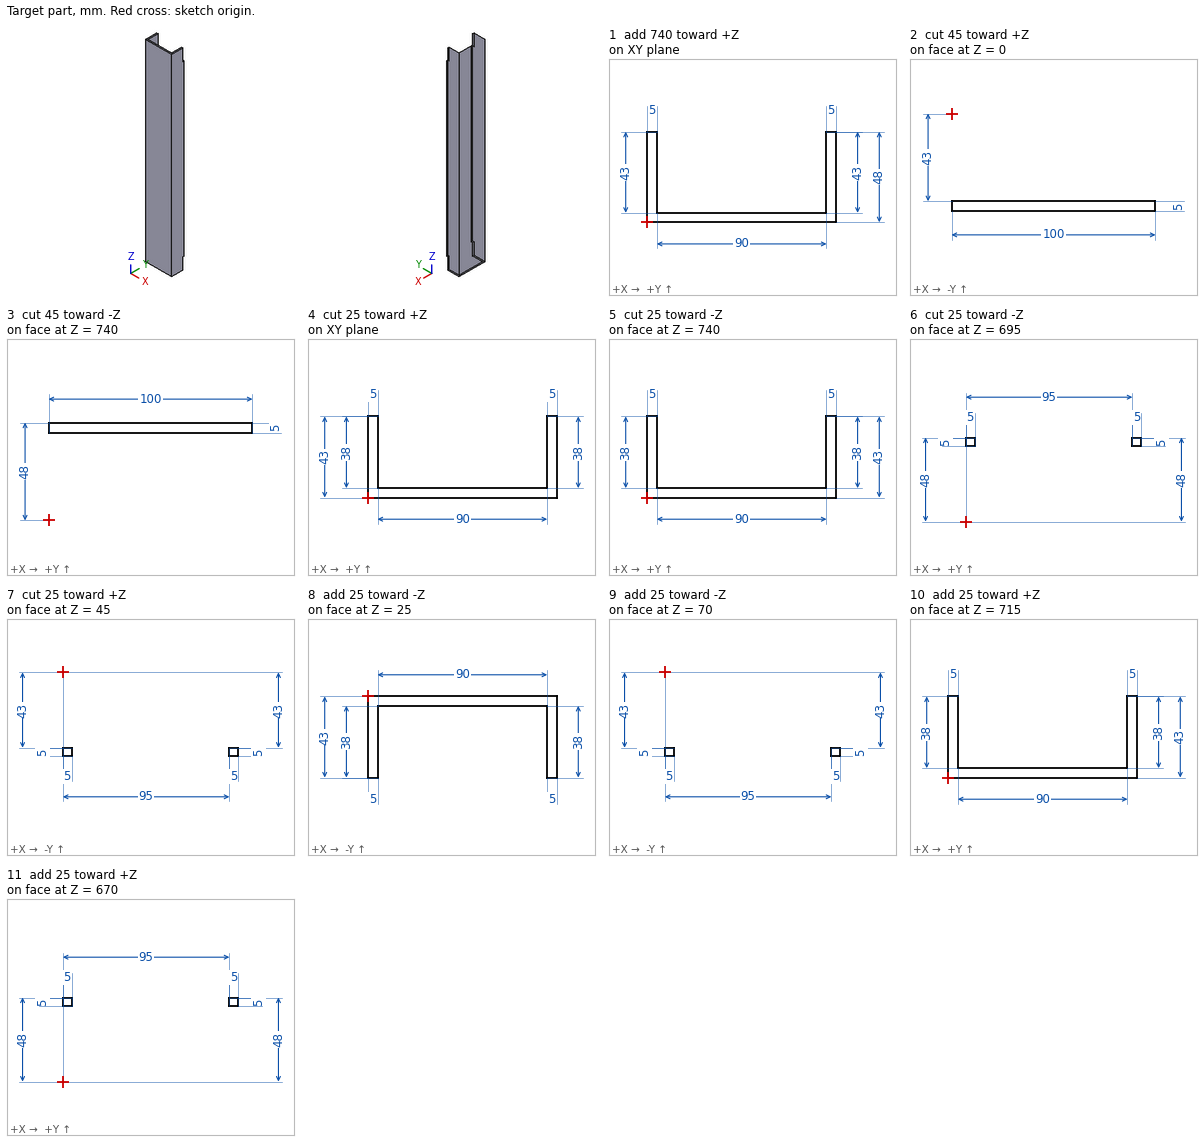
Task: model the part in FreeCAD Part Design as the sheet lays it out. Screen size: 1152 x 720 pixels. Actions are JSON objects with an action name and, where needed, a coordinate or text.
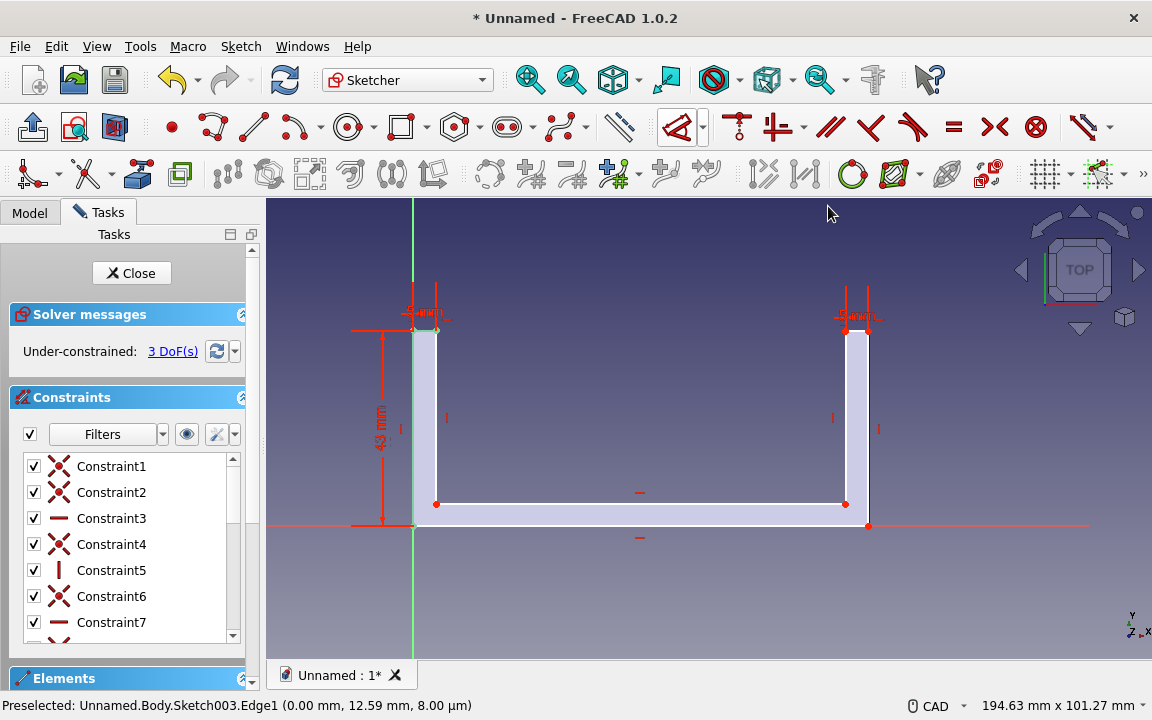
{"action": "left_click", "coordinate": [436, 383]}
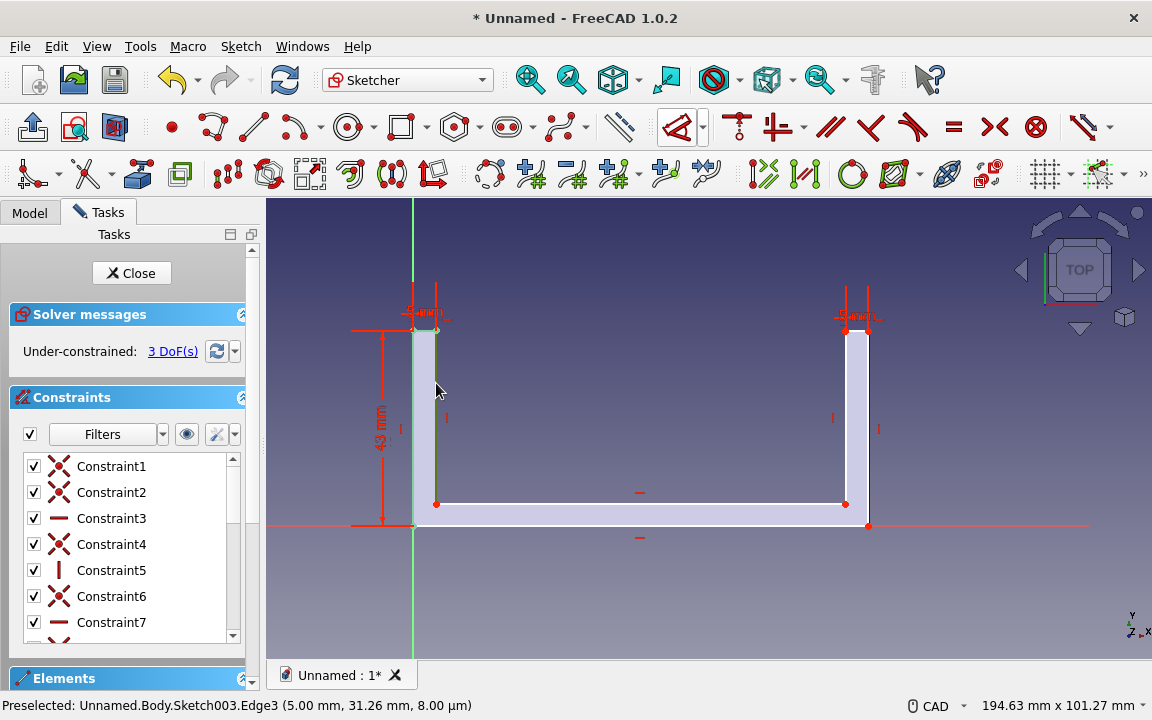
{"action": "left_click", "coordinate": [702, 128]}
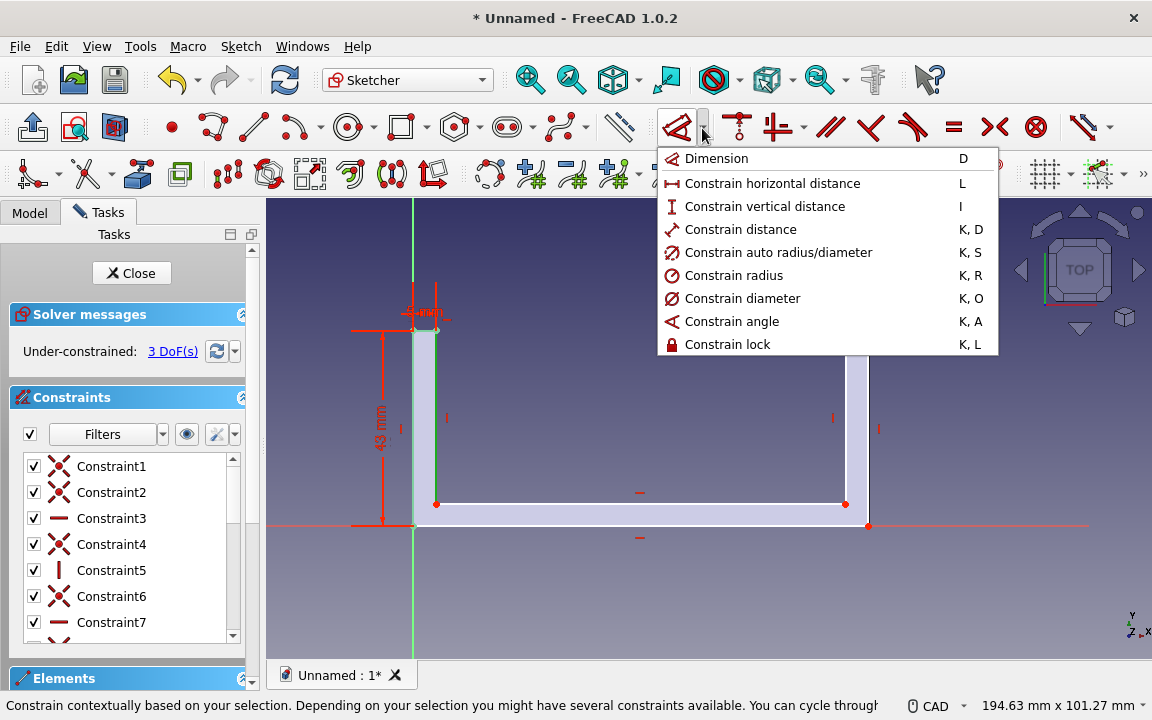
{"action": "left_click", "coordinate": [828, 206]}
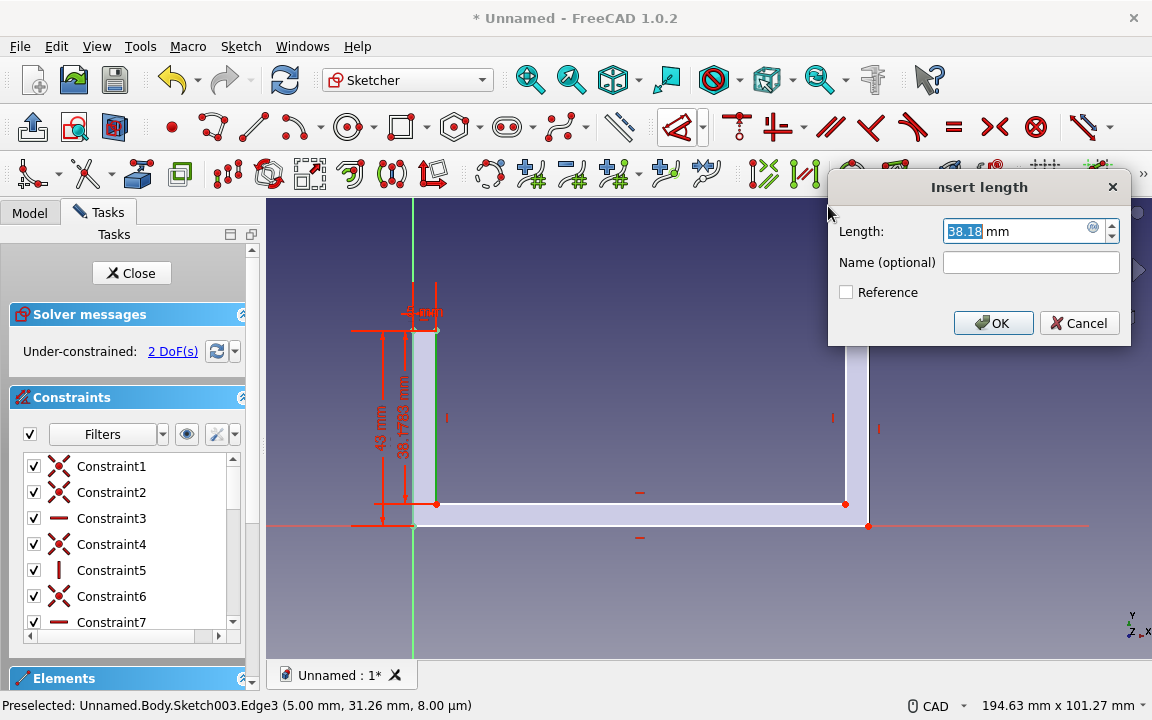
{"action": "type", "text": "38"}
{"action": "key", "text": "Return"}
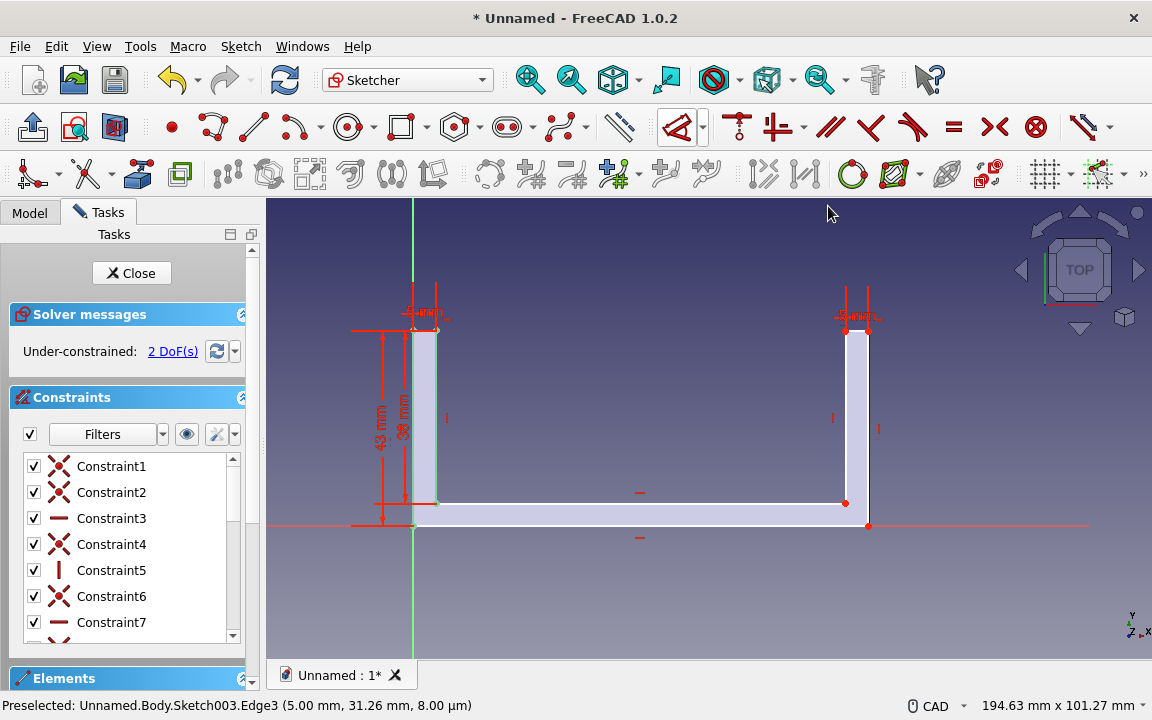
{"action": "left_click", "coordinate": [559, 504]}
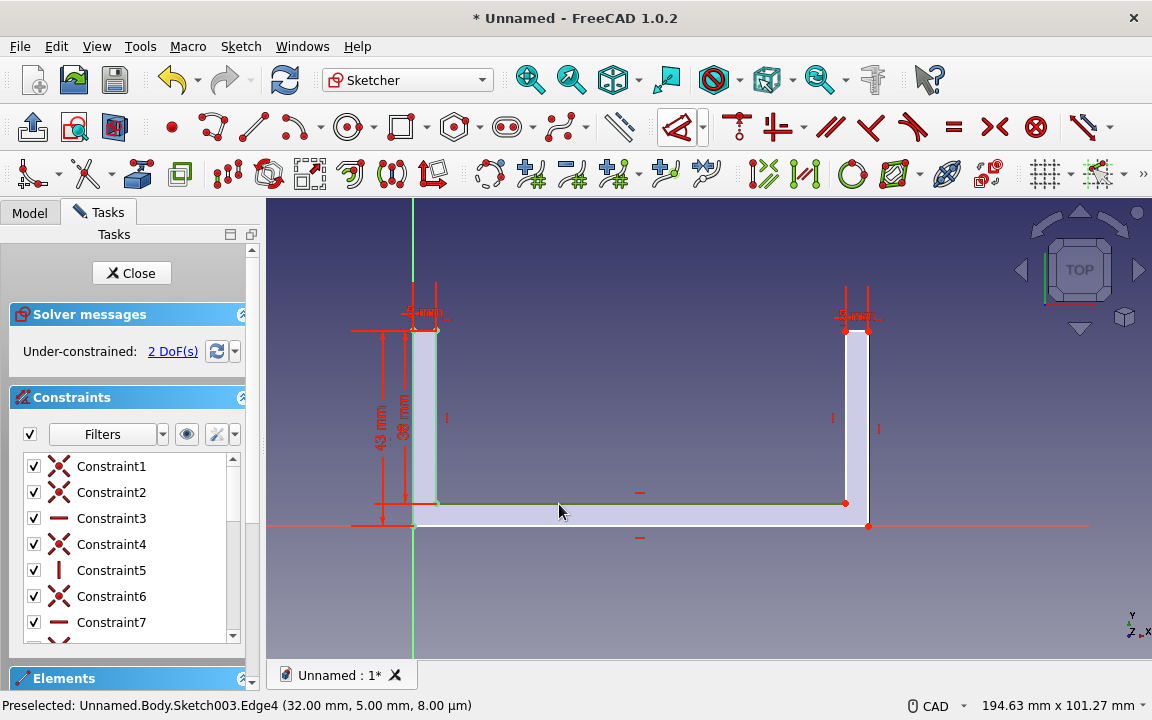
{"action": "left_click", "coordinate": [702, 128]}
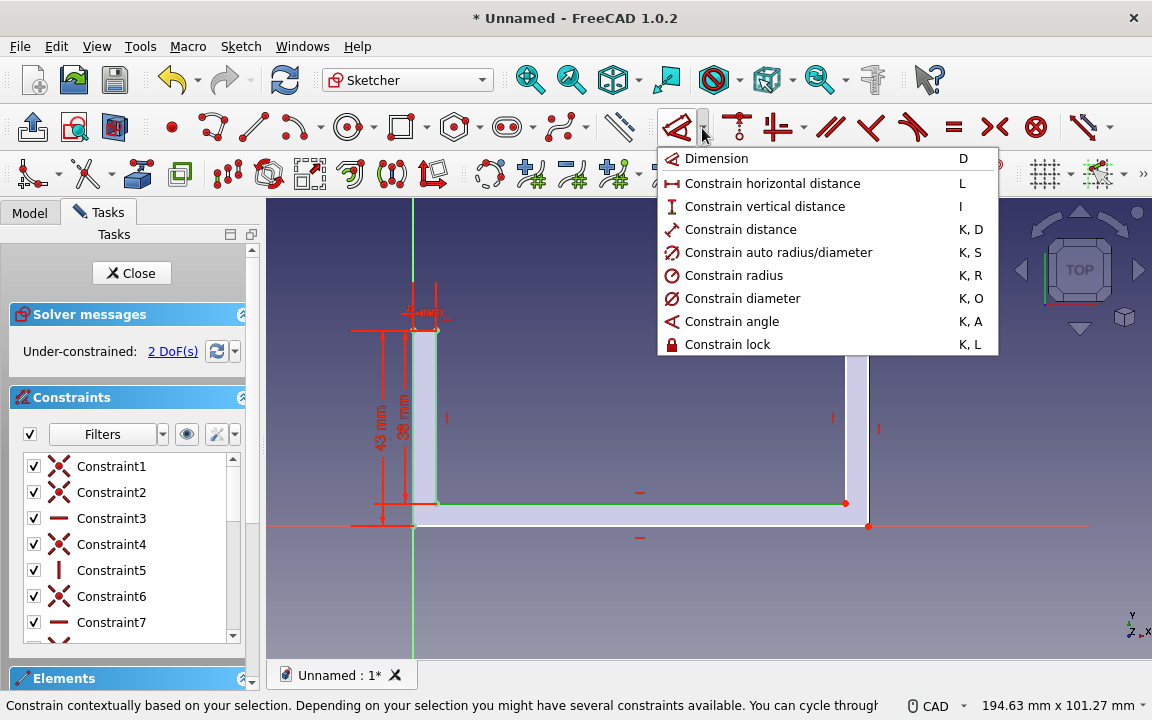
{"action": "left_click", "coordinate": [828, 184]}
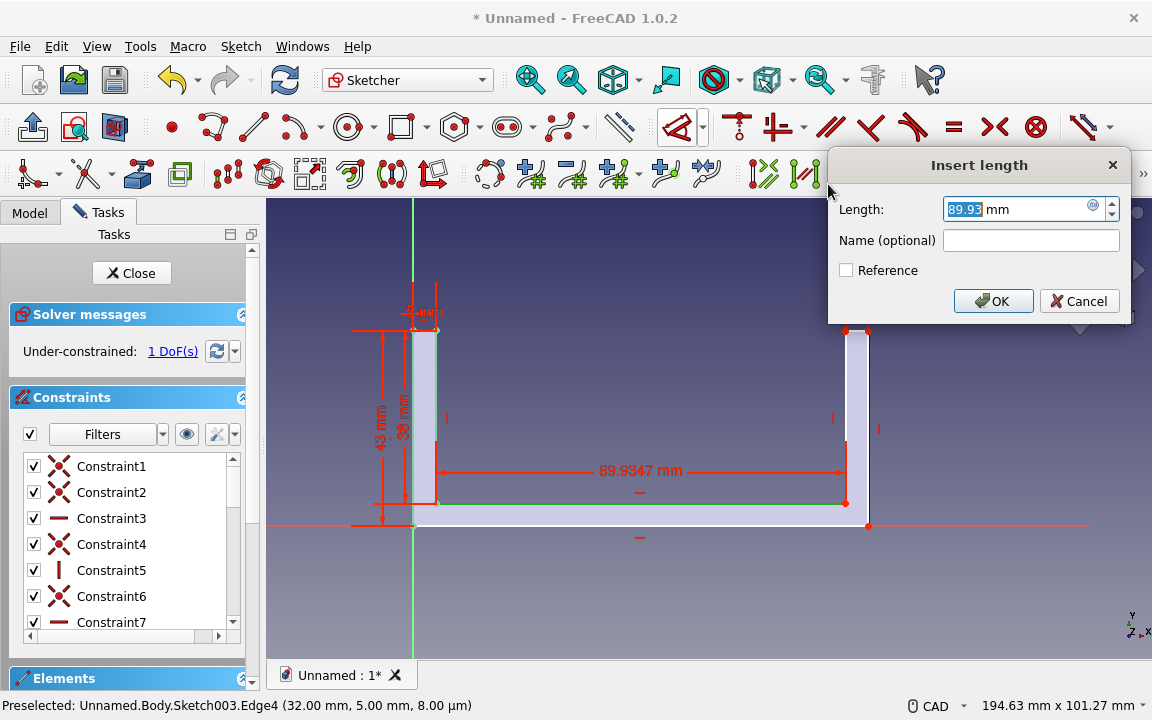
{"action": "type", "text": "90"}
{"action": "key", "text": "Return"}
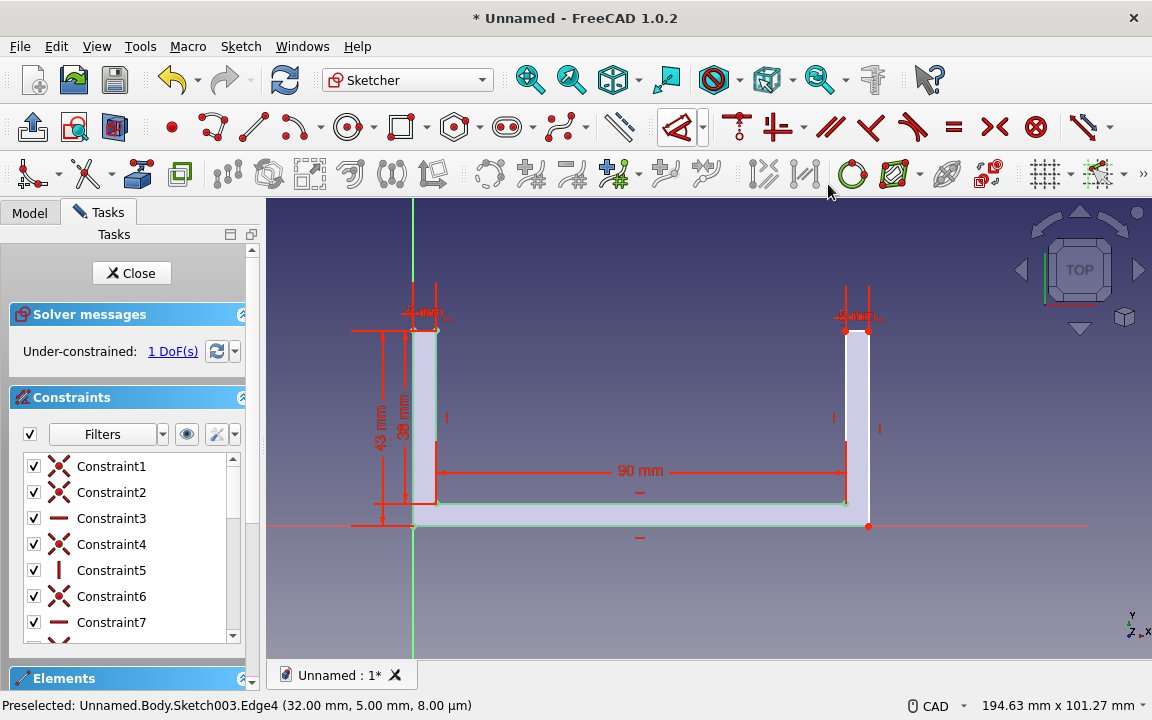
{"action": "left_click", "coordinate": [846, 452]}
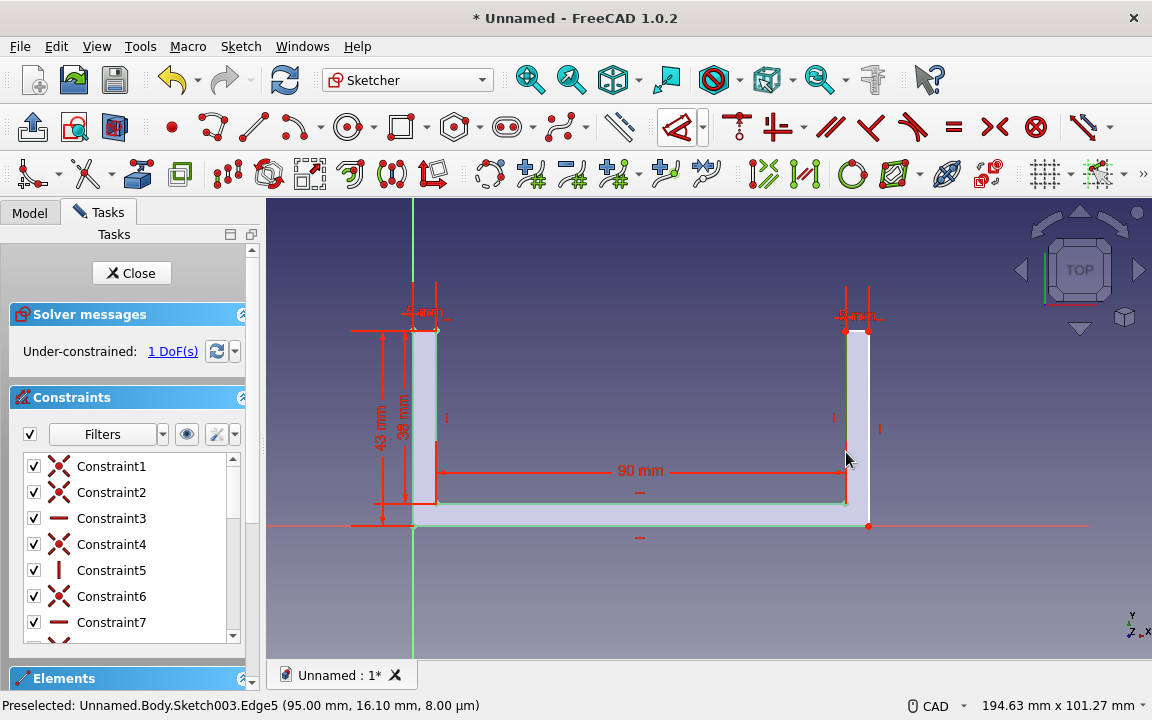
{"action": "left_click", "coordinate": [702, 128]}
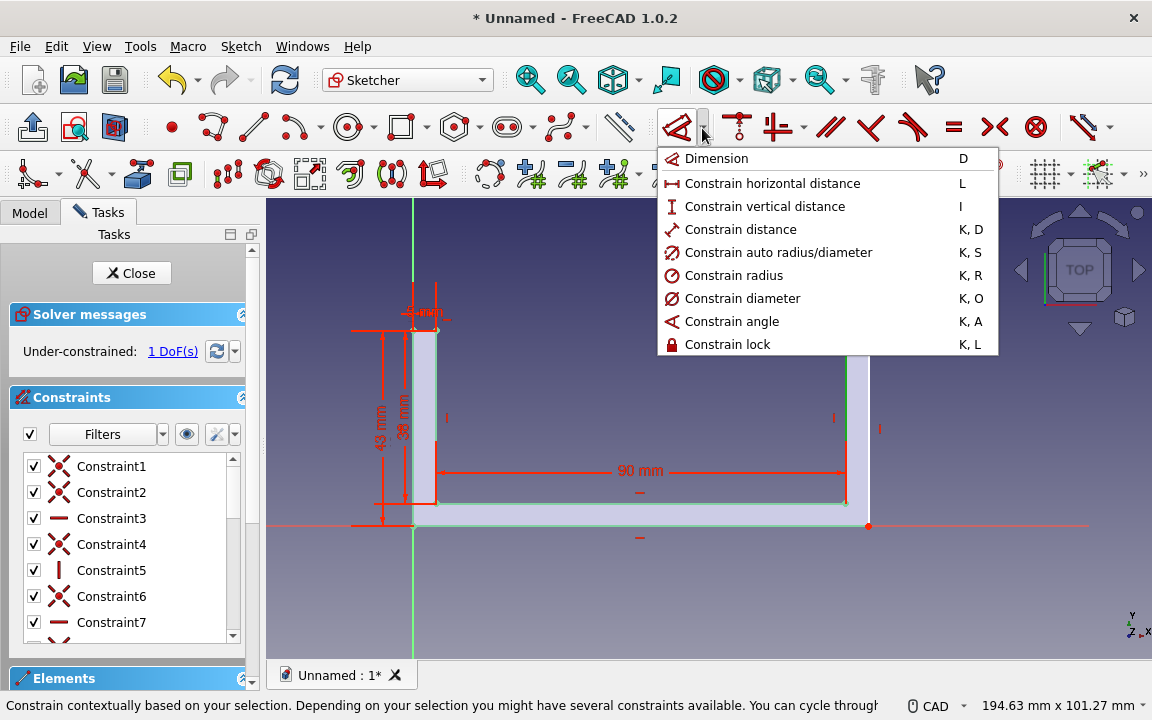
{"action": "left_click", "coordinate": [828, 206]}